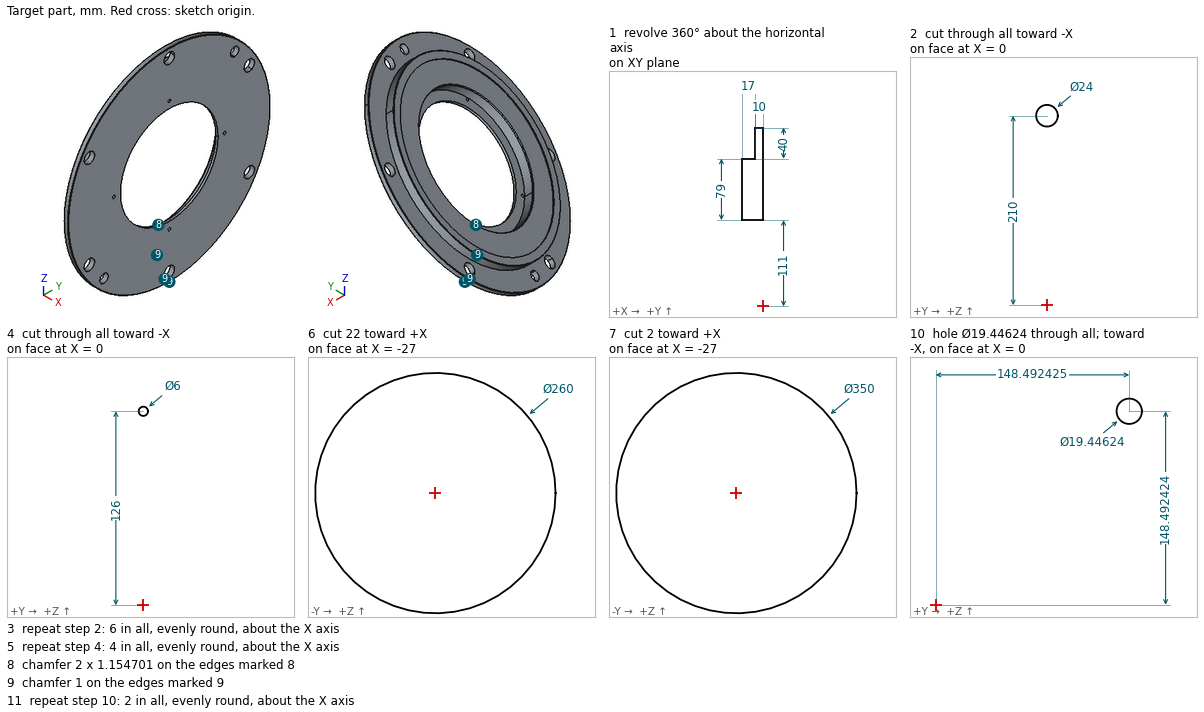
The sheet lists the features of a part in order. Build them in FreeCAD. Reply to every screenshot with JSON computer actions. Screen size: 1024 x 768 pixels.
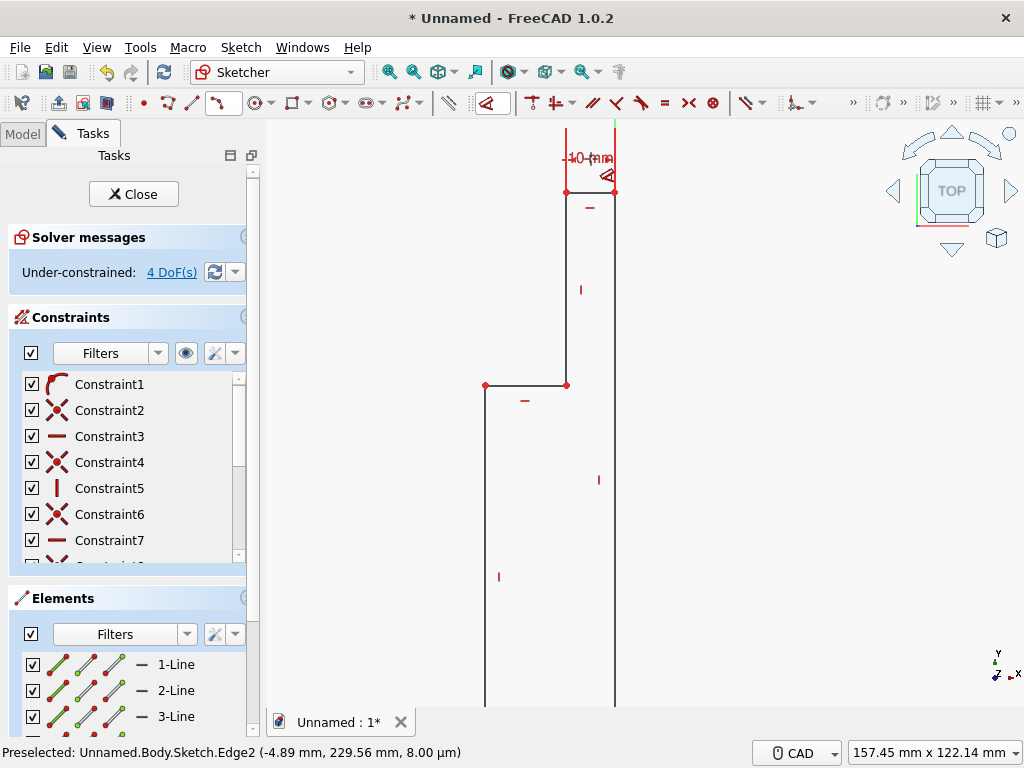
{"action": "left_click", "coordinate": [566, 251]}
{"action": "left_click", "coordinate": [600, 289]}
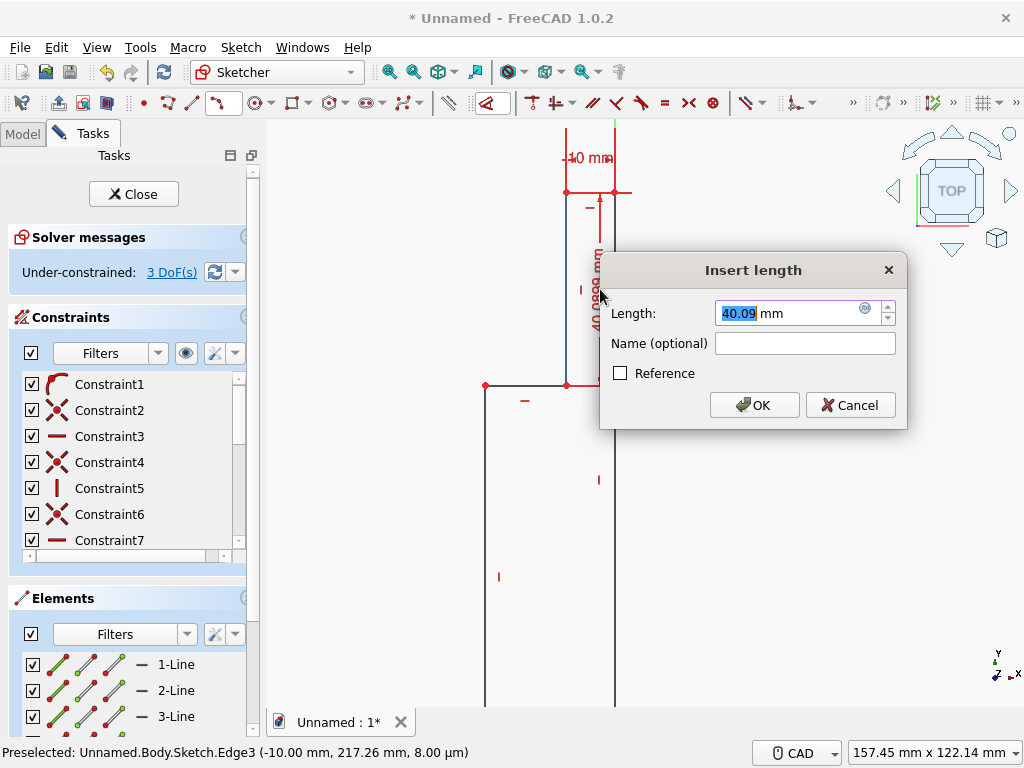
{"action": "type", "text": "40"}
{"action": "key", "text": "Return"}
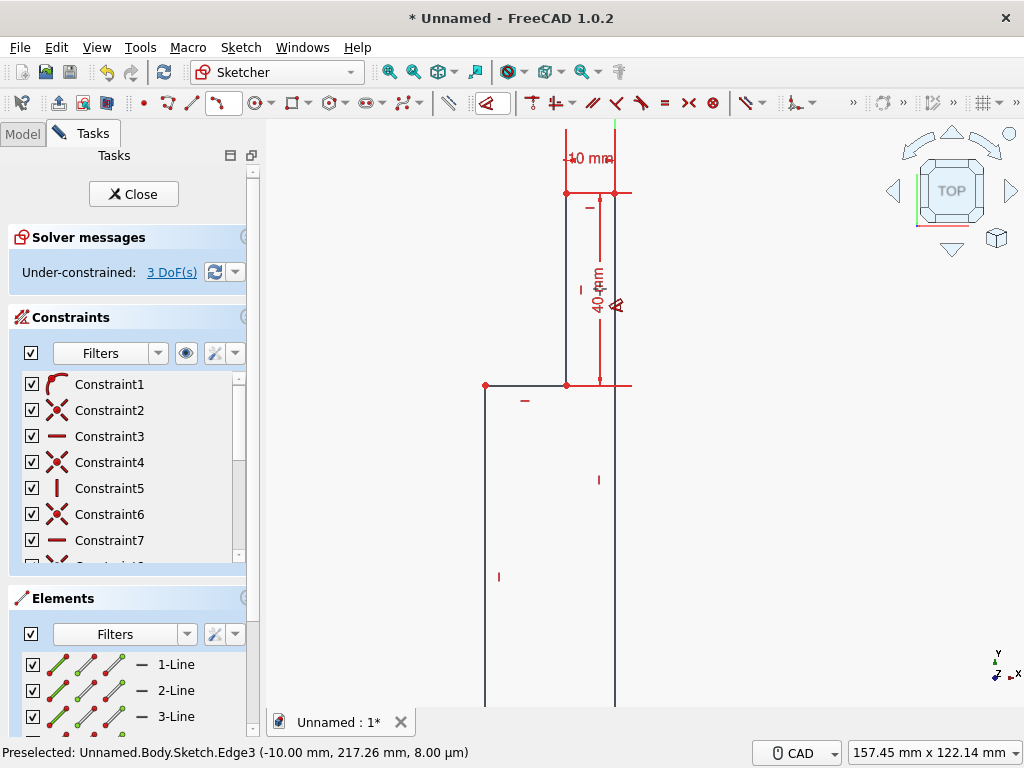
{"action": "left_click", "coordinate": [542, 386]}
{"action": "left_click", "coordinate": [526, 352]}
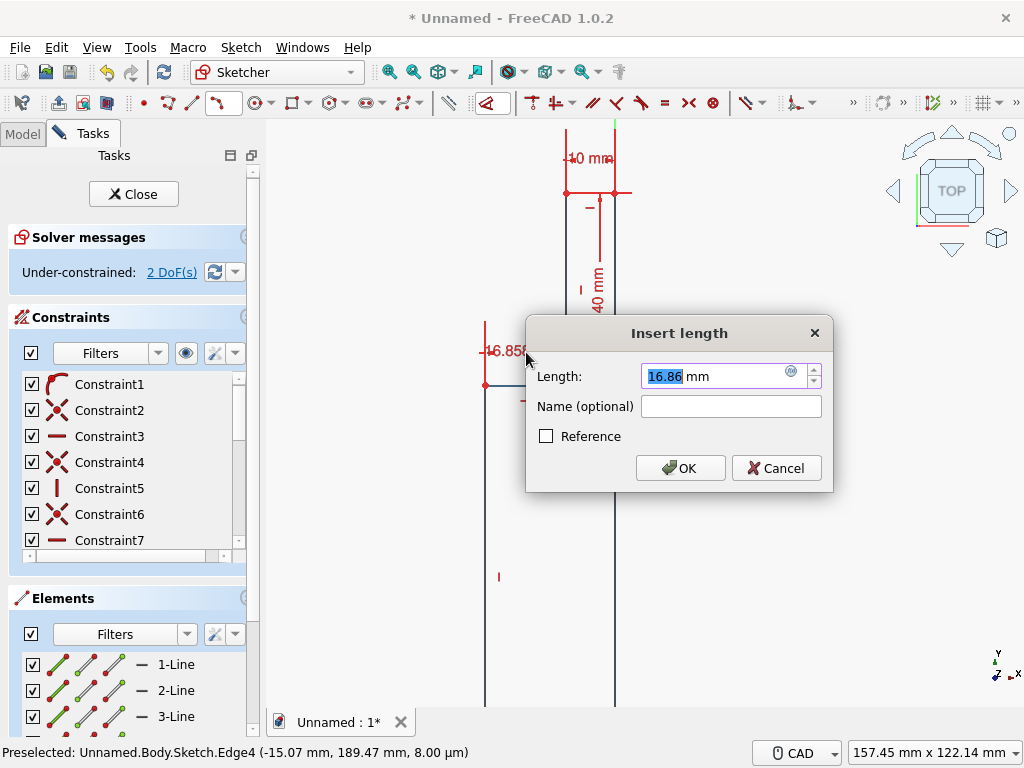
{"action": "type", "text": "17"}
{"action": "key", "text": "Return"}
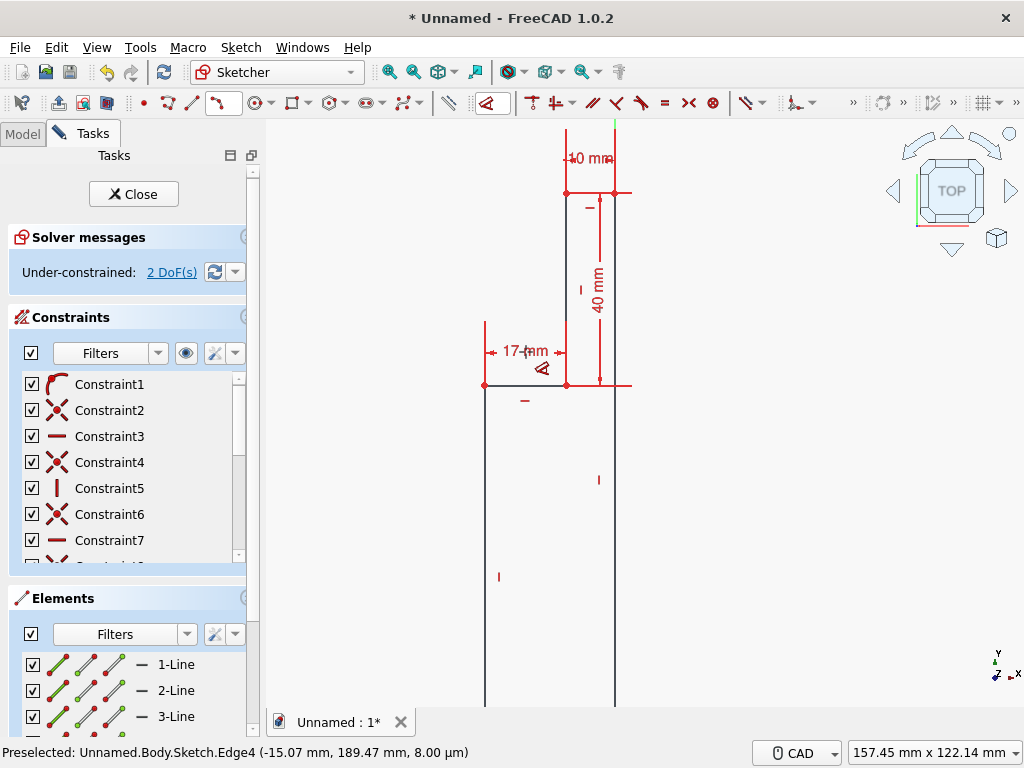
{"action": "left_click", "coordinate": [485, 500]}
{"action": "left_click", "coordinate": [451, 532]}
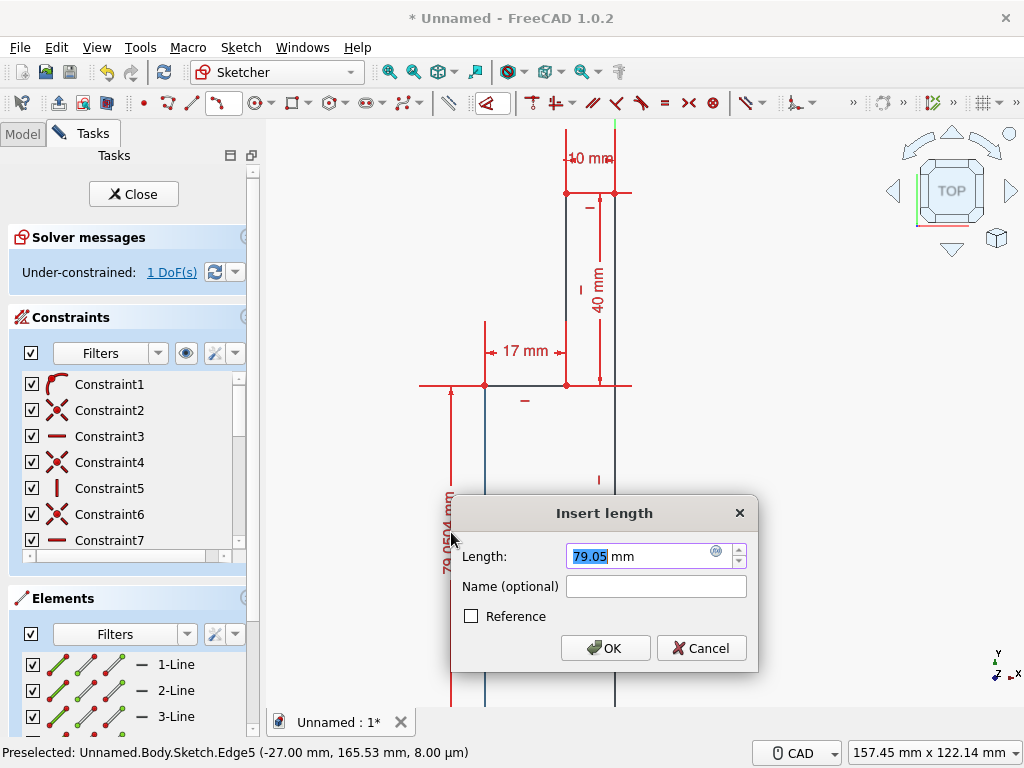
{"action": "type", "text": "79"}
{"action": "key", "text": "Return"}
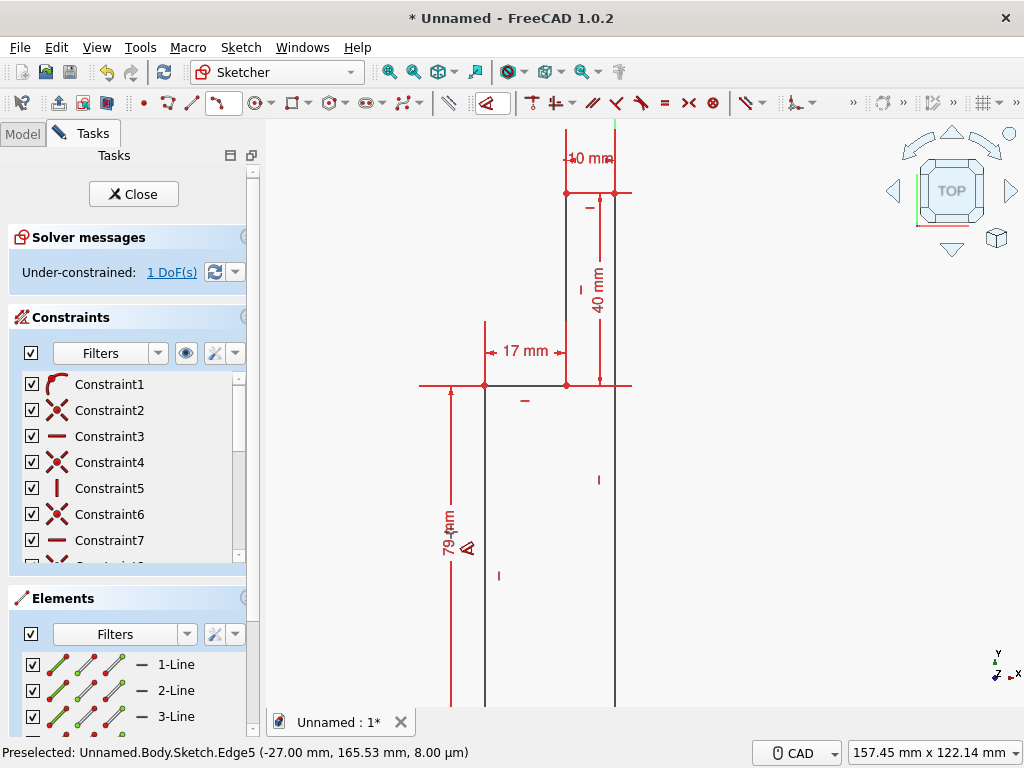
{"action": "scroll", "coordinate": [592, 220], "scroll_direction": "down", "scroll_amount": 5}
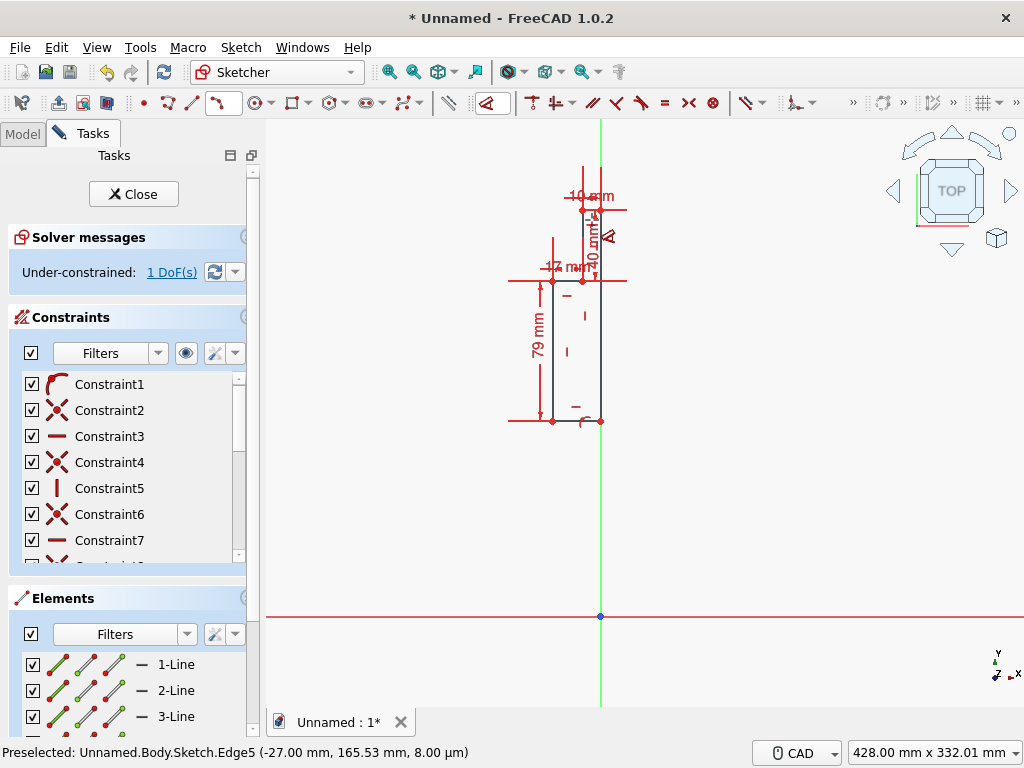
{"action": "left_click", "coordinate": [601, 421]}
{"action": "left_click", "coordinate": [635, 519]}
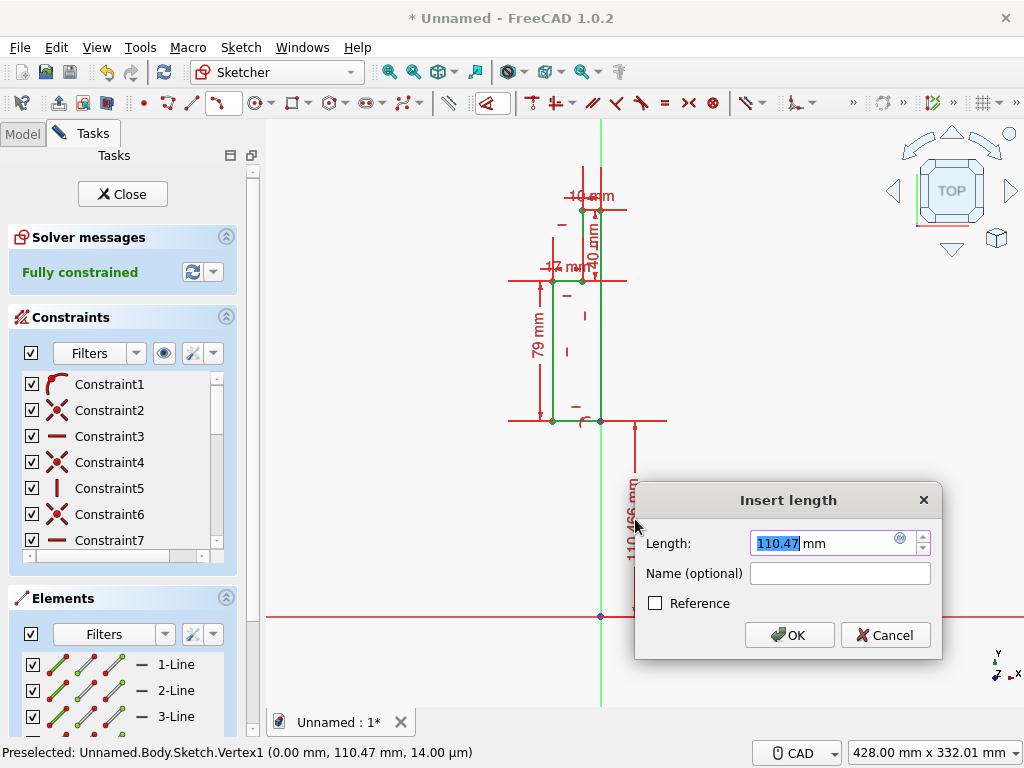
{"action": "type", "text": "111"}
{"action": "key", "text": "Return"}
{"action": "key", "text": "Escape"}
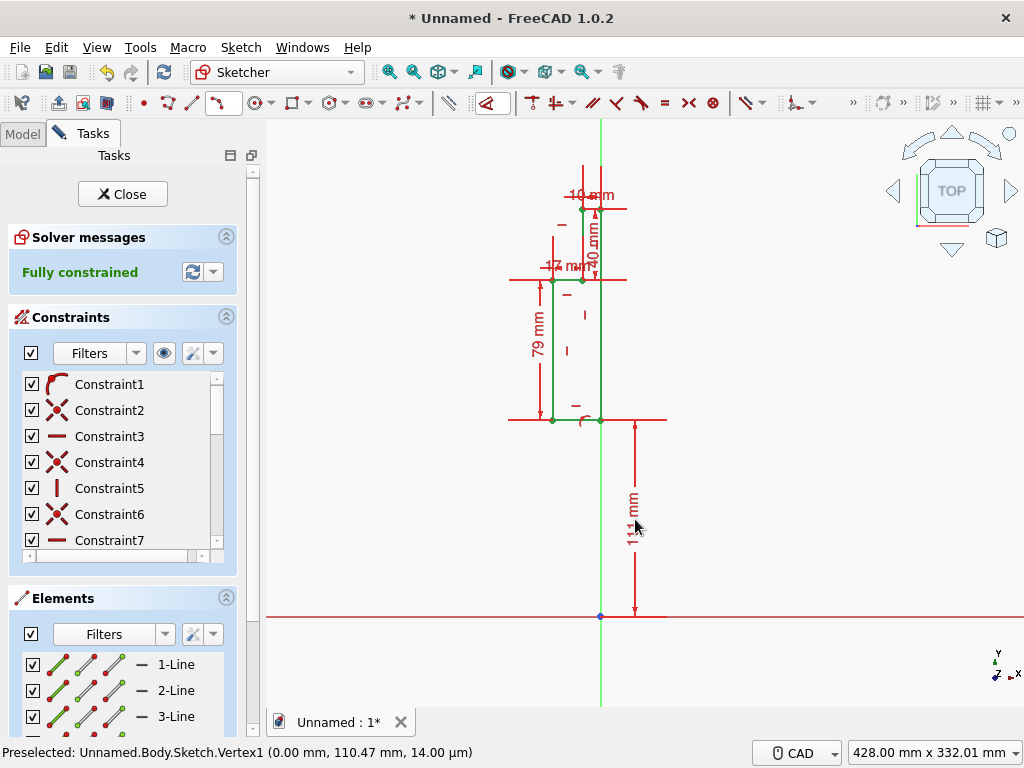
{"action": "left_click", "coordinate": [123, 194]}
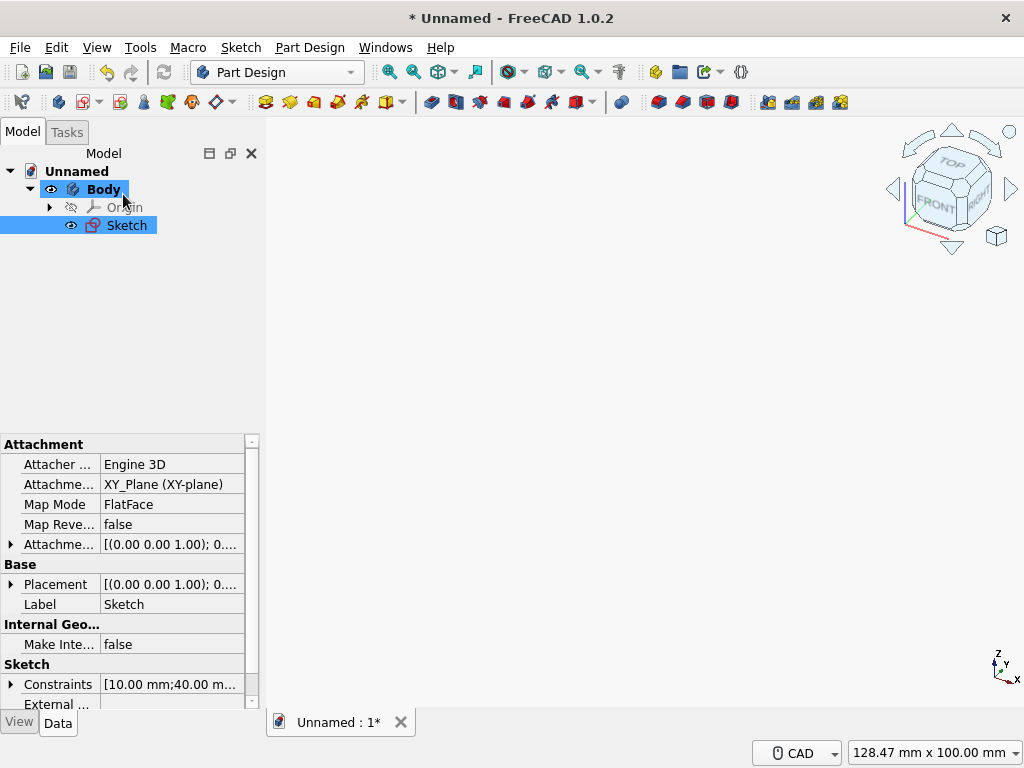
{"action": "left_click", "coordinate": [290, 102]}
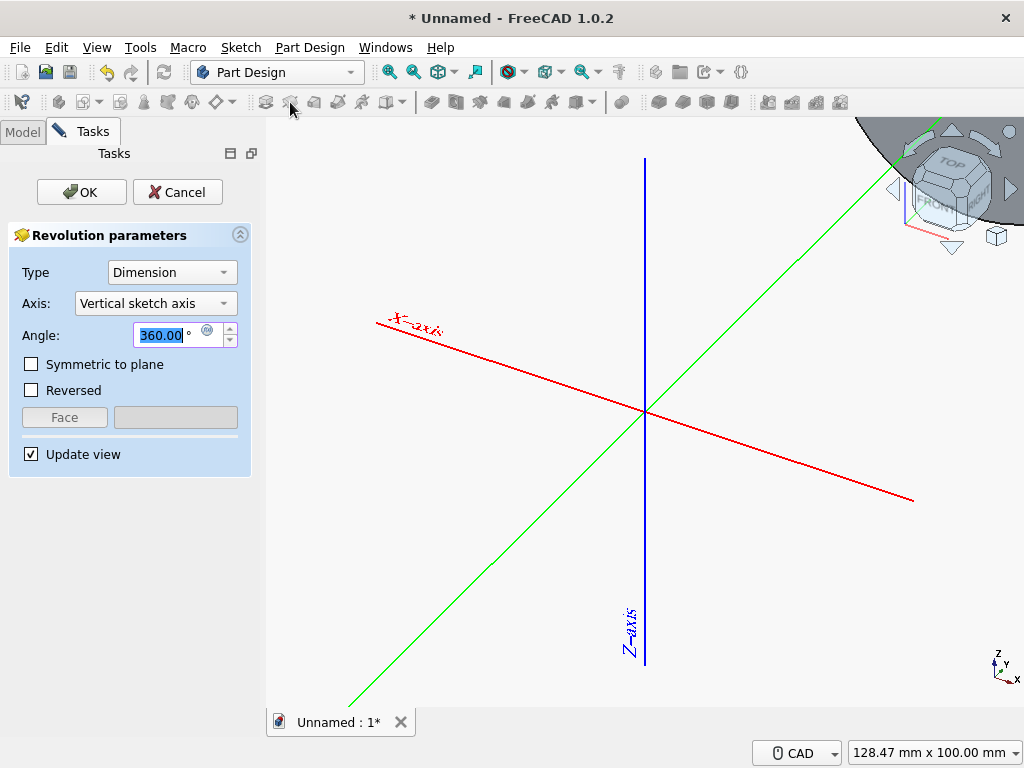
{"action": "left_click", "coordinate": [156, 304]}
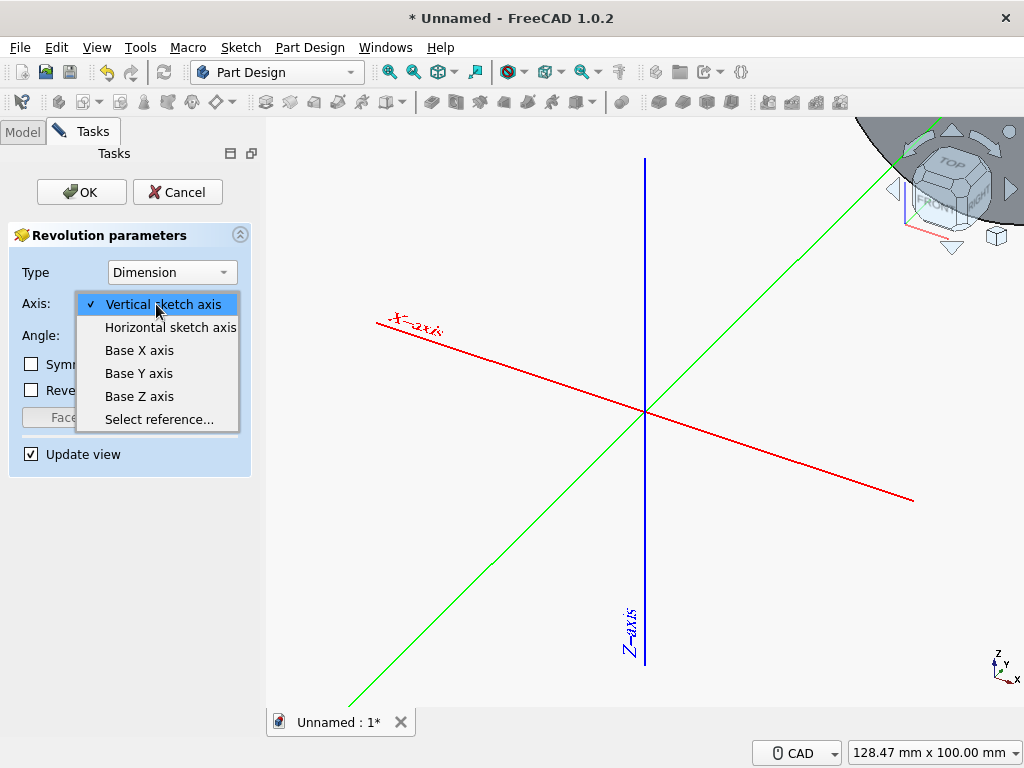
{"action": "left_click", "coordinate": [156, 328]}